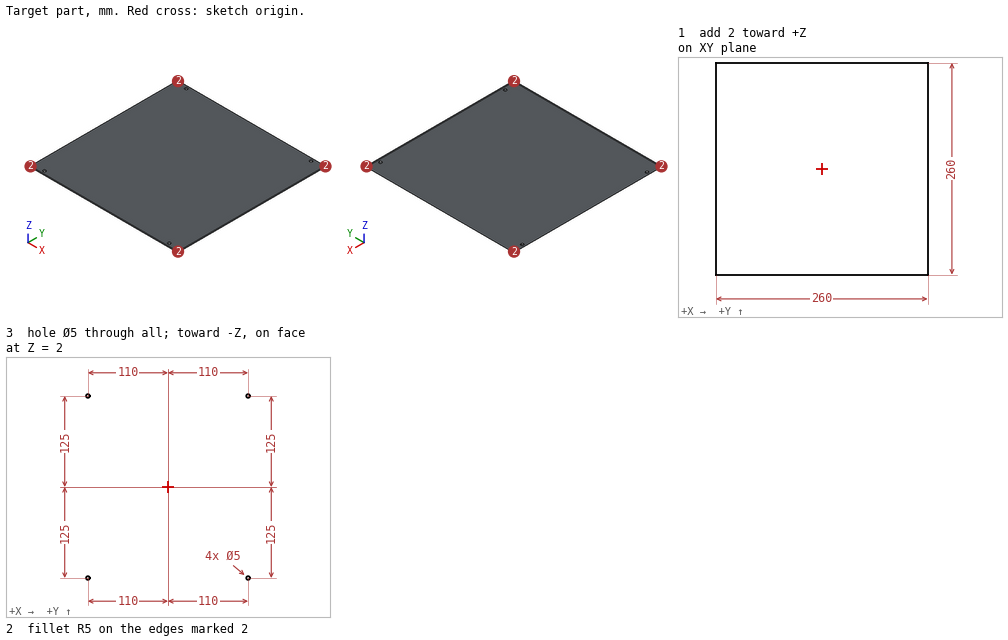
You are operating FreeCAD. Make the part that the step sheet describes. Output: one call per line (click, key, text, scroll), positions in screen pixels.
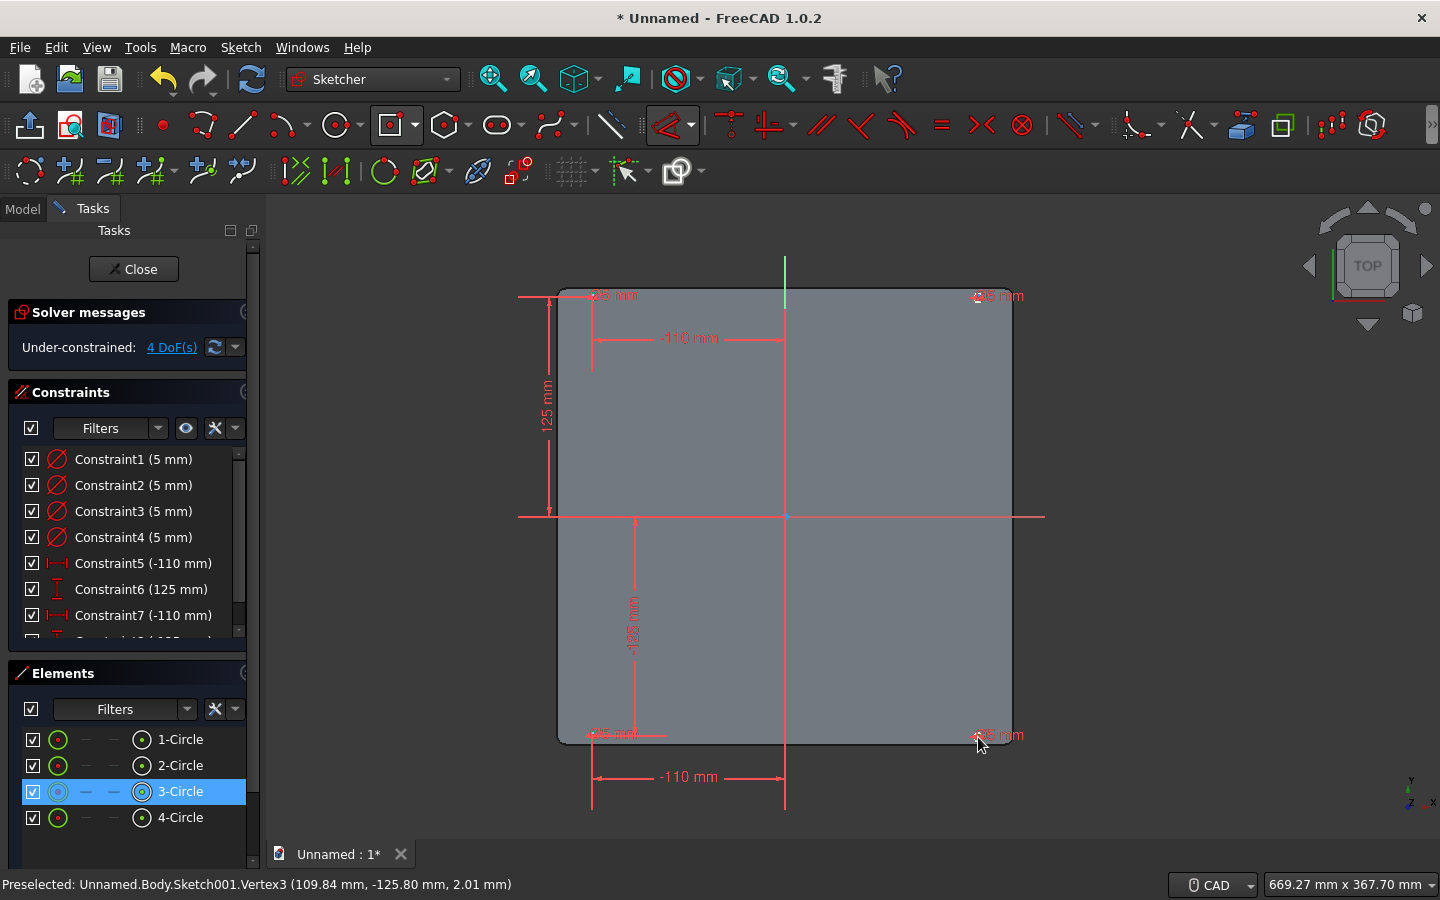
key(l)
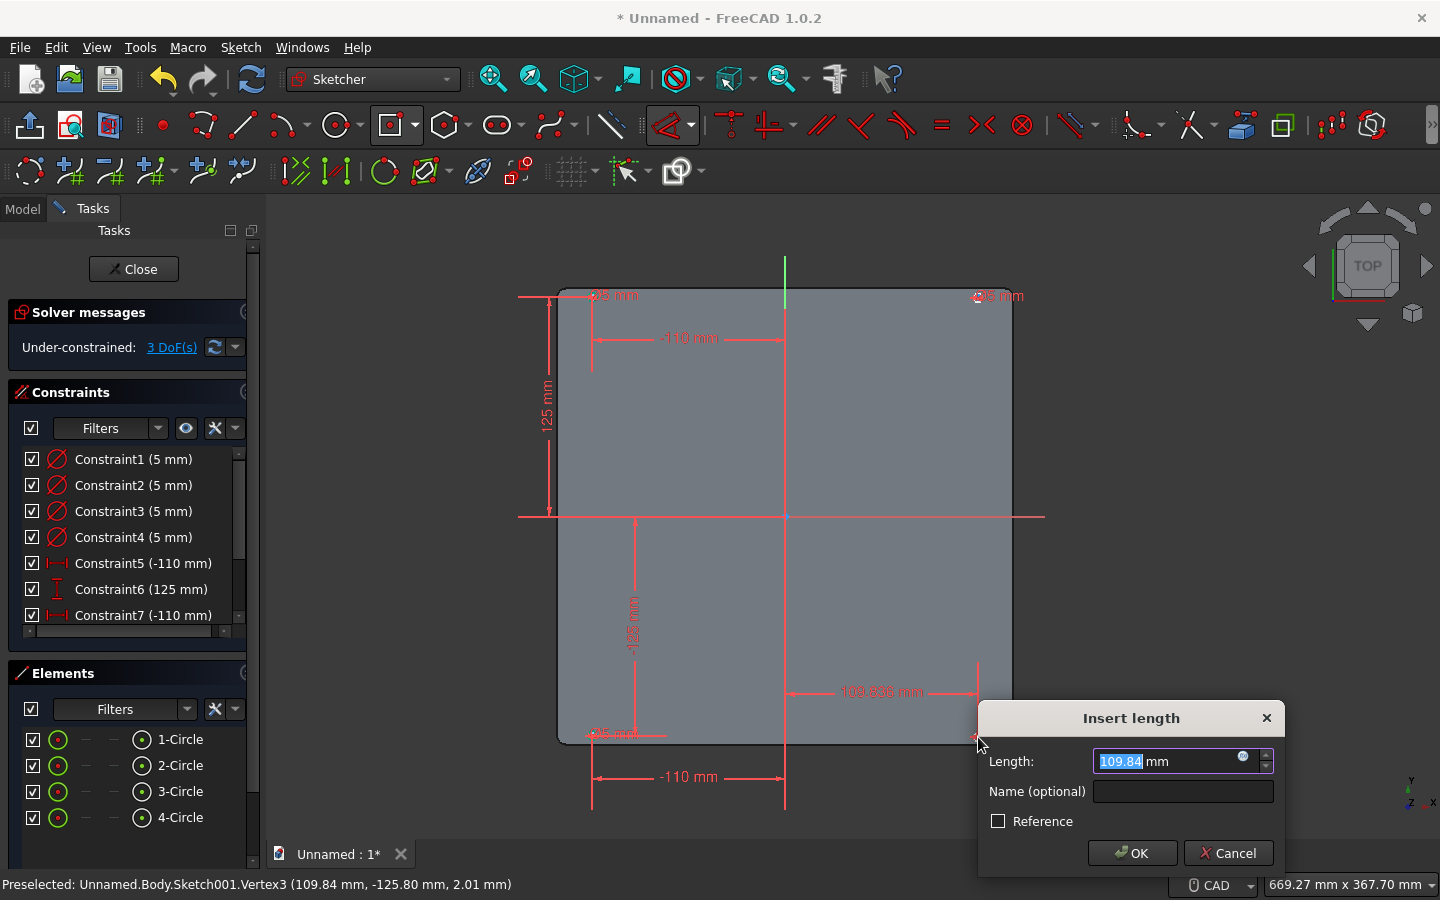
text(110)
key(Return)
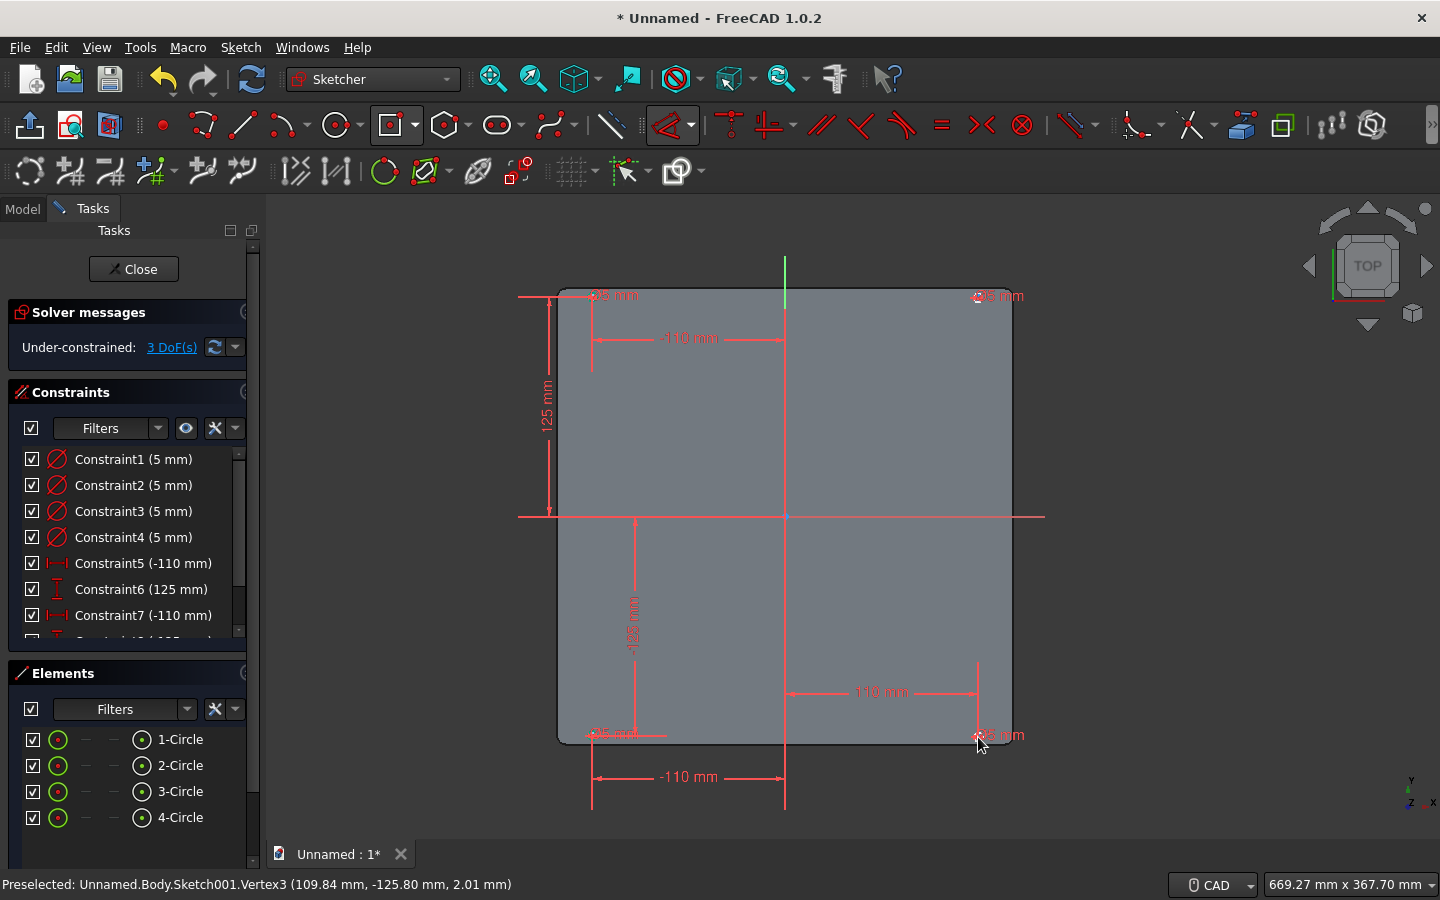
click(978, 737)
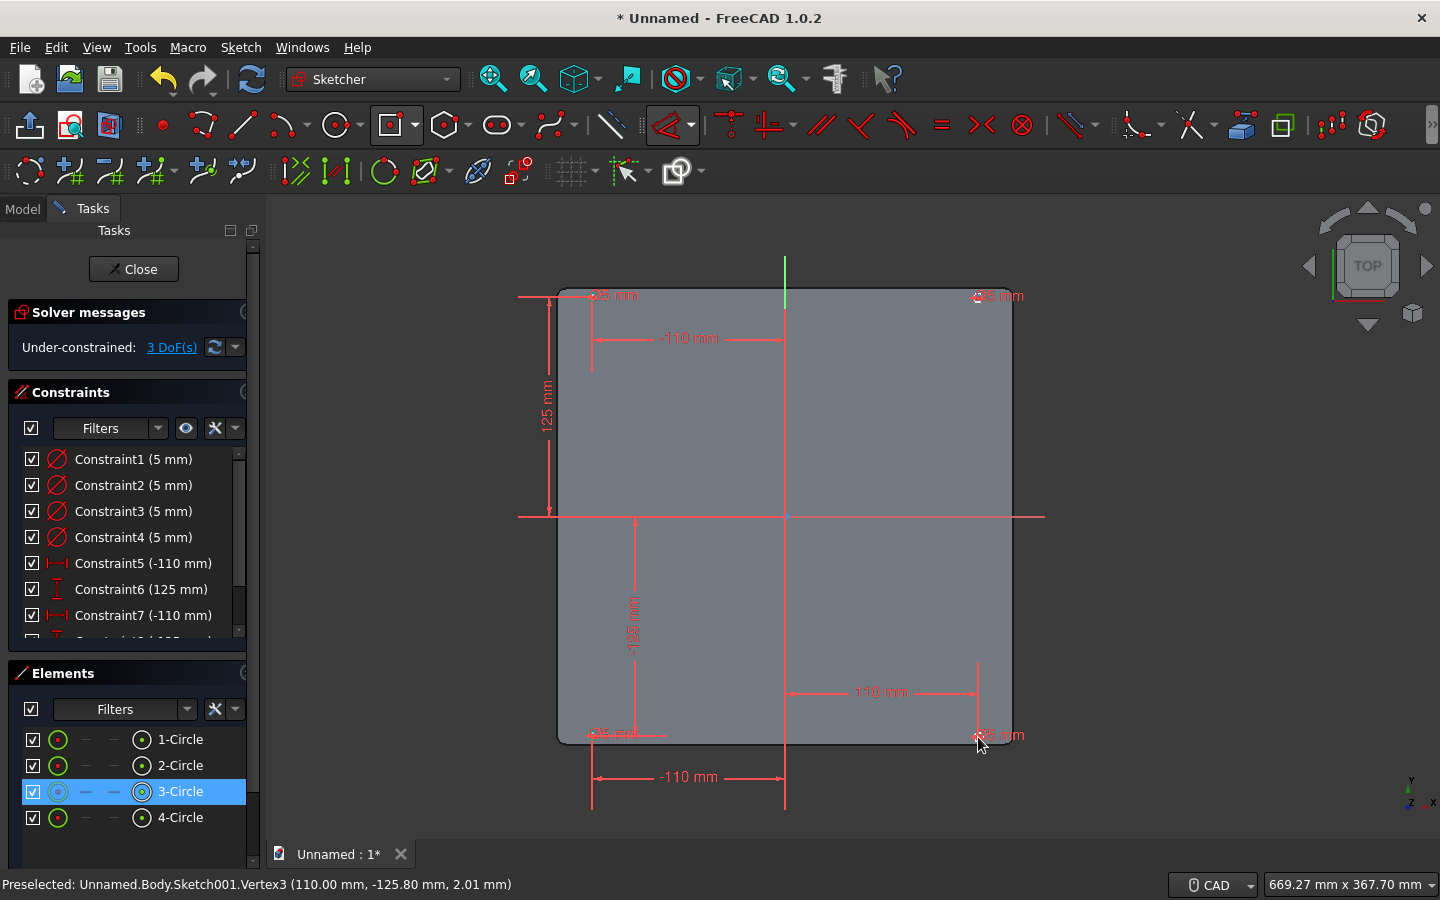
click(694, 126)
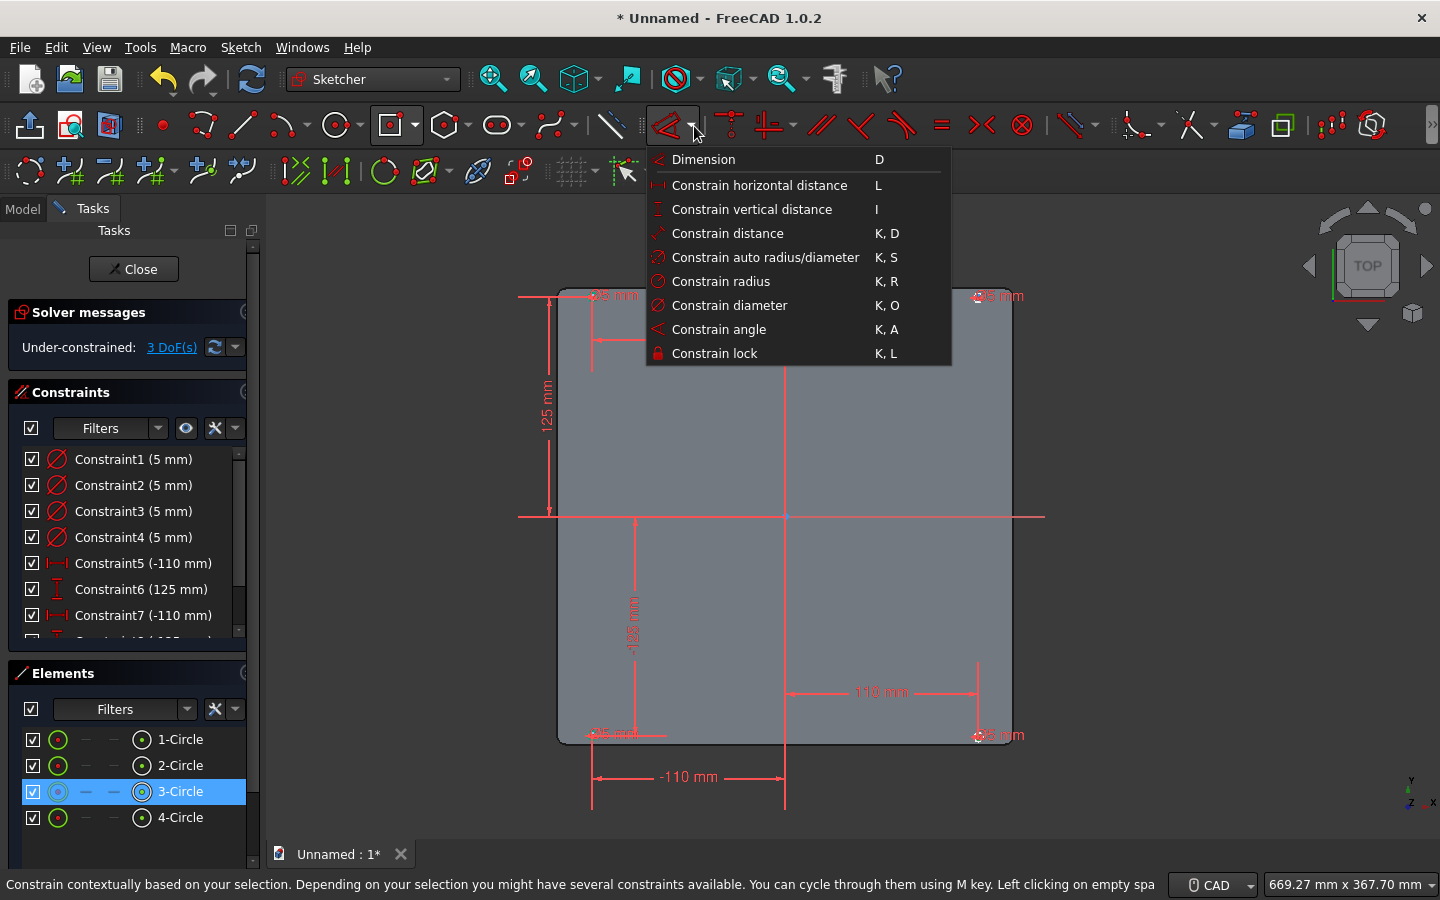
click(799, 209)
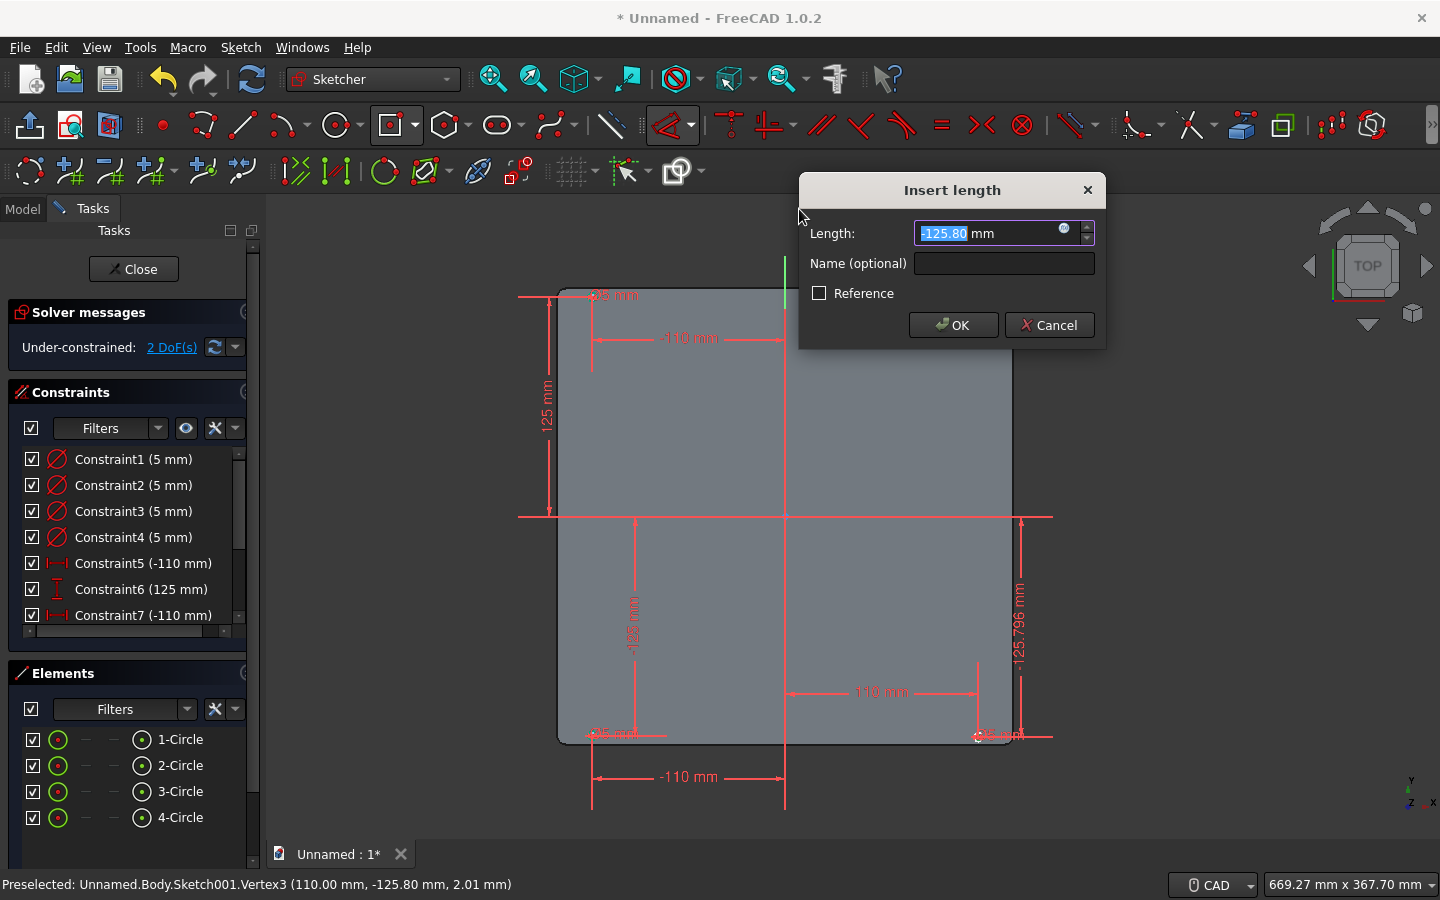
text(-125)
key(Return)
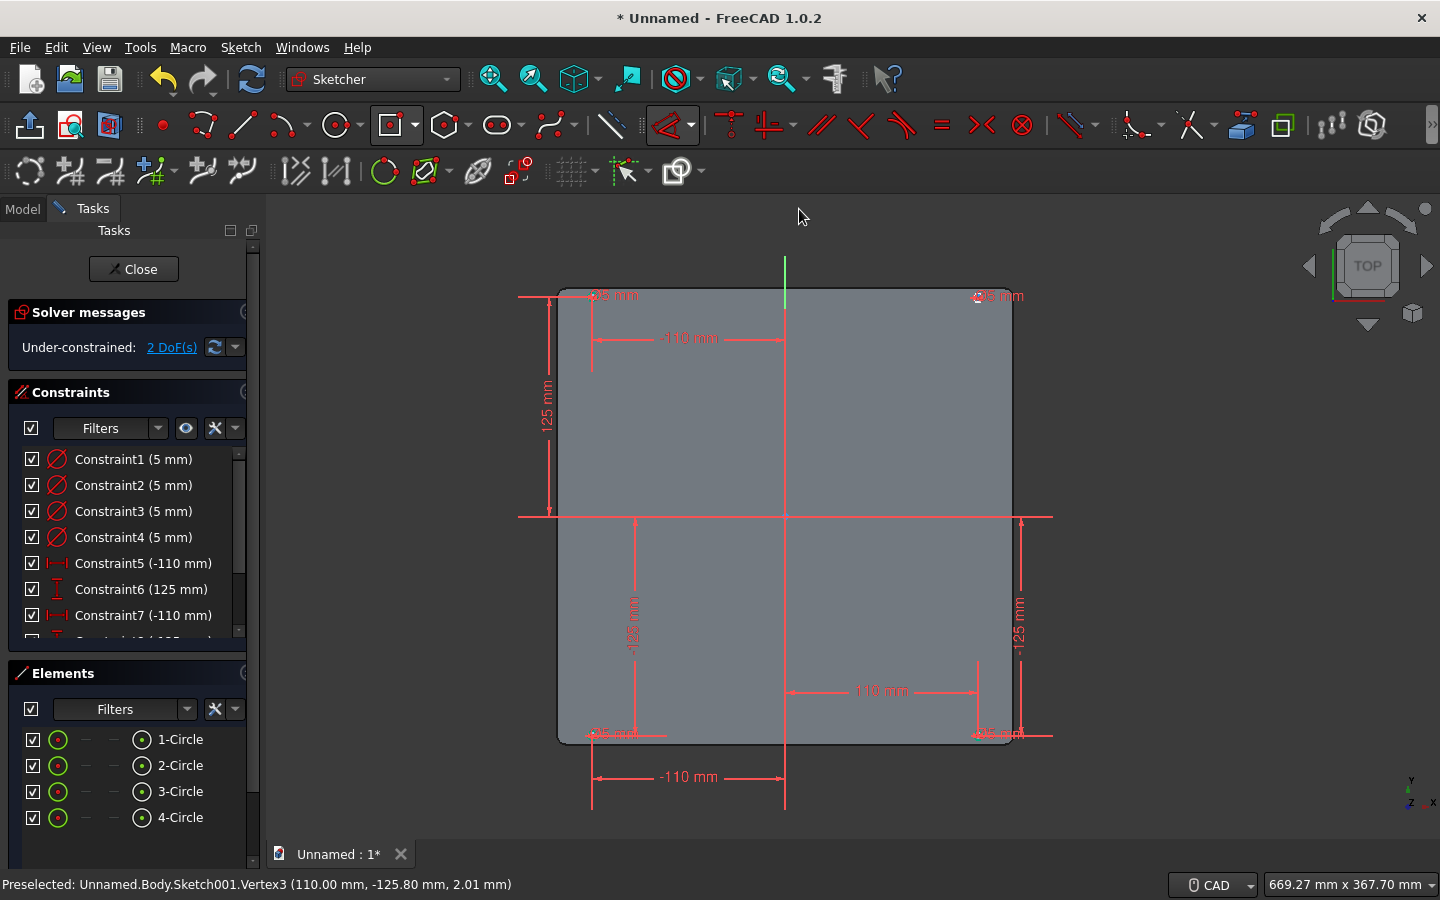
click(978, 298)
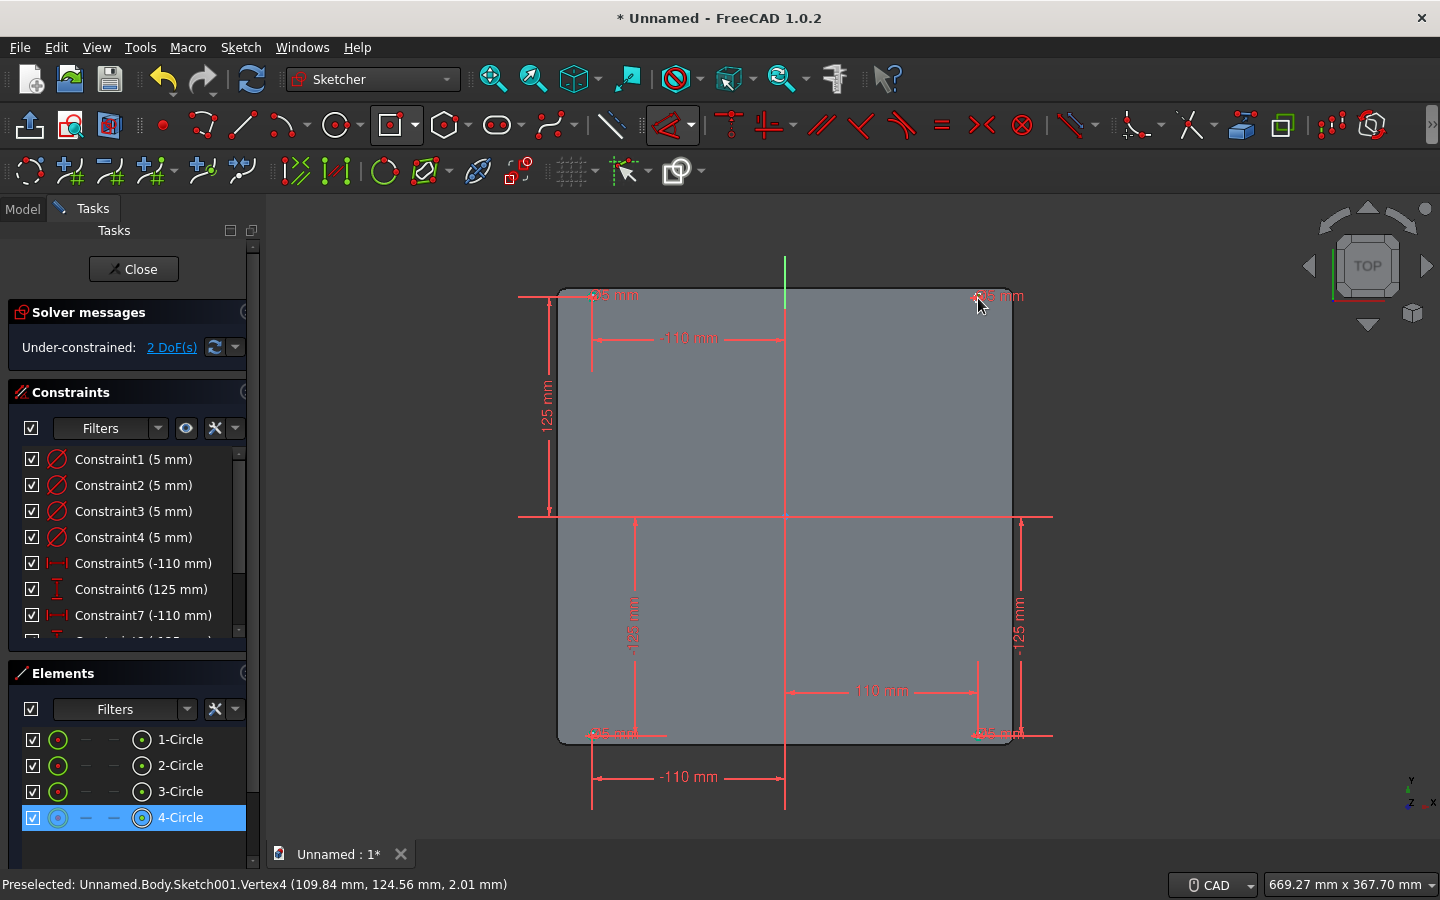
key(l)